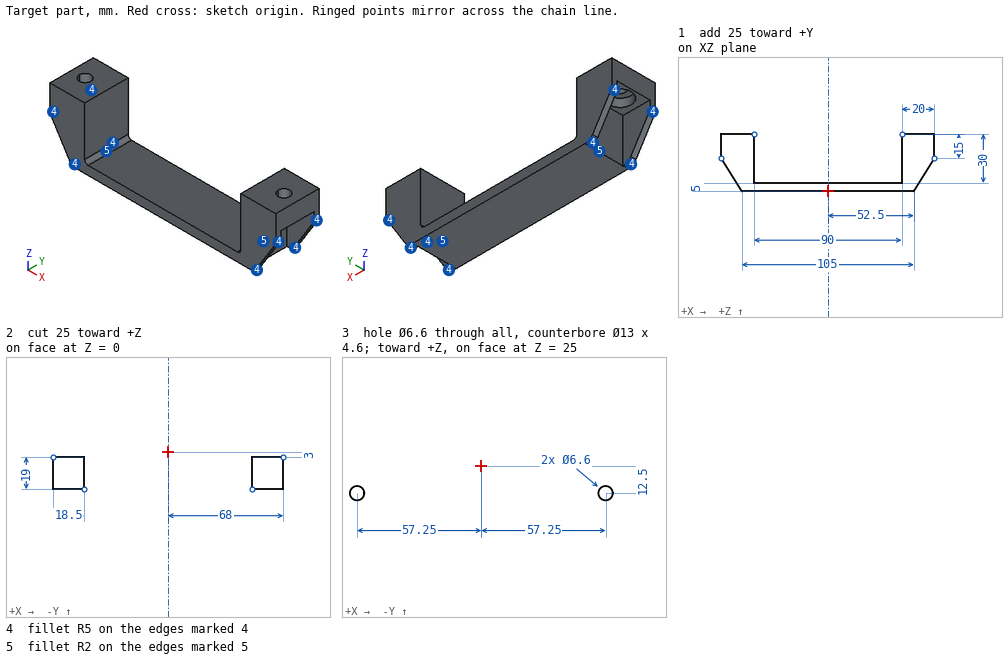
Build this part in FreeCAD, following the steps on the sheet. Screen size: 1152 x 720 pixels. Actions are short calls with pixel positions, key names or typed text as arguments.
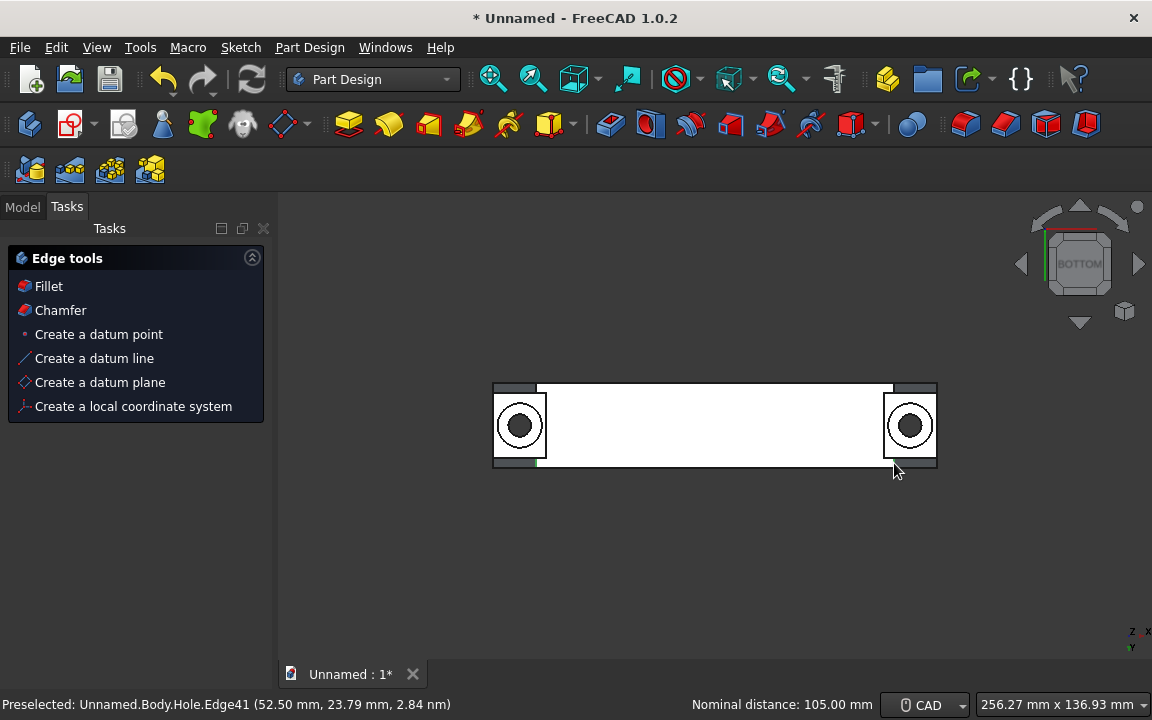
click(894, 388, ctrl)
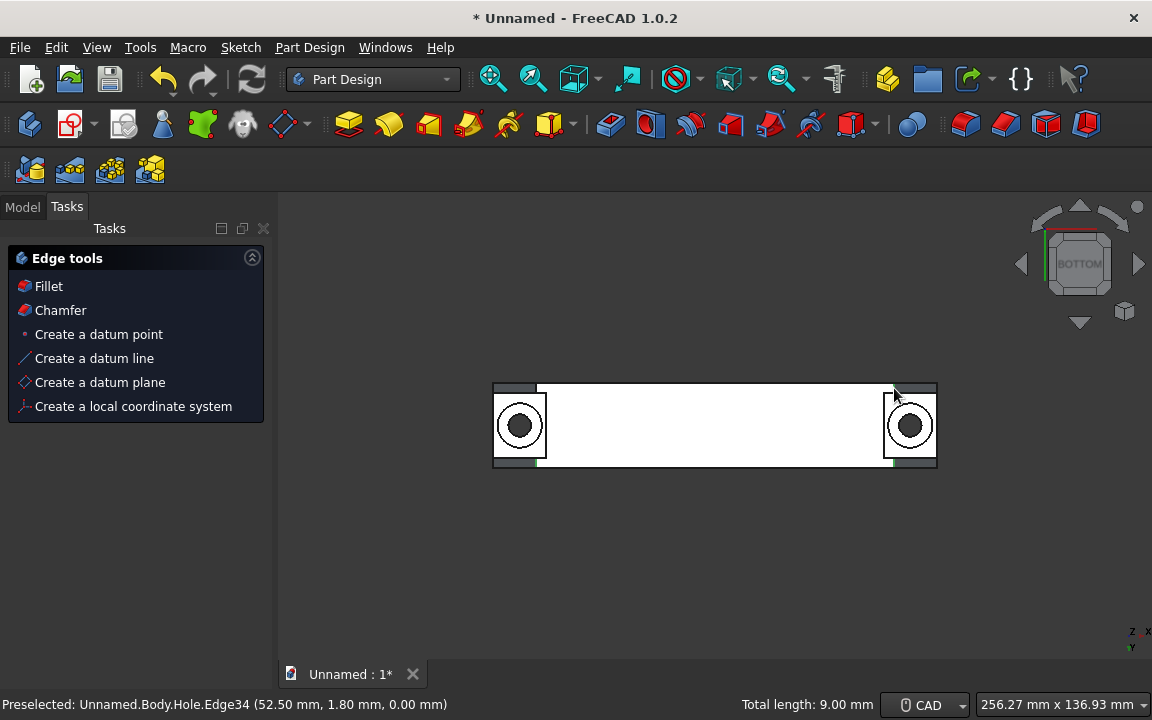
click(536, 388, ctrl)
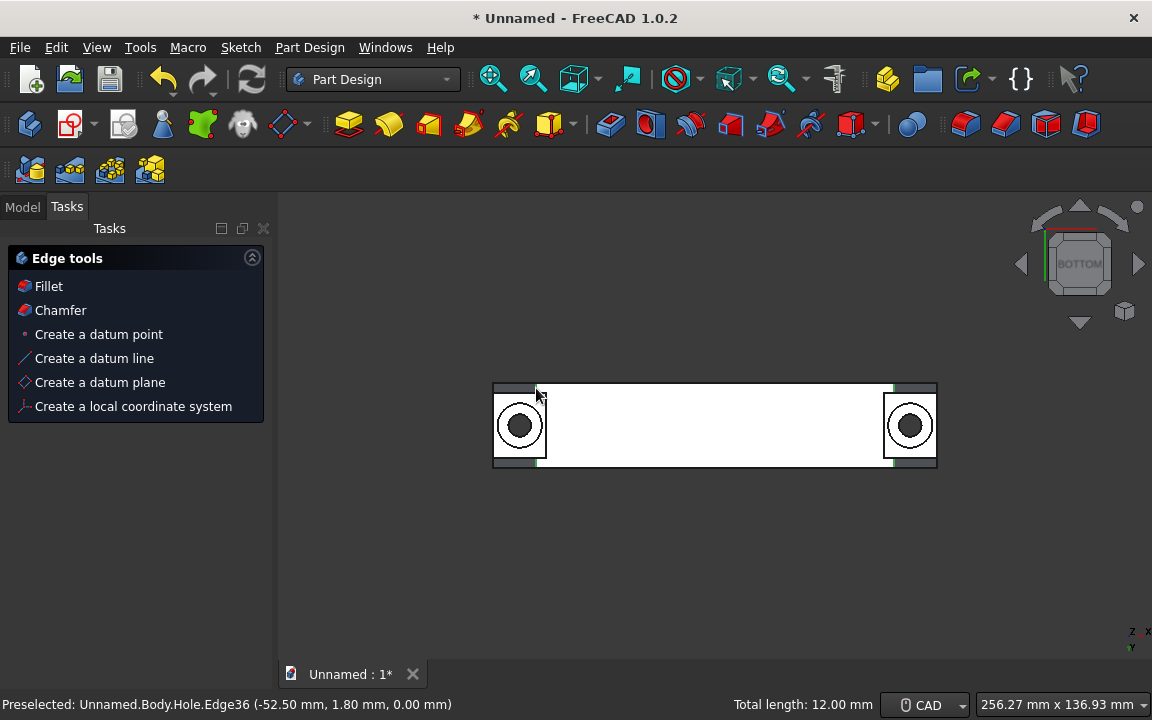
scroll(937, 462, up, 7)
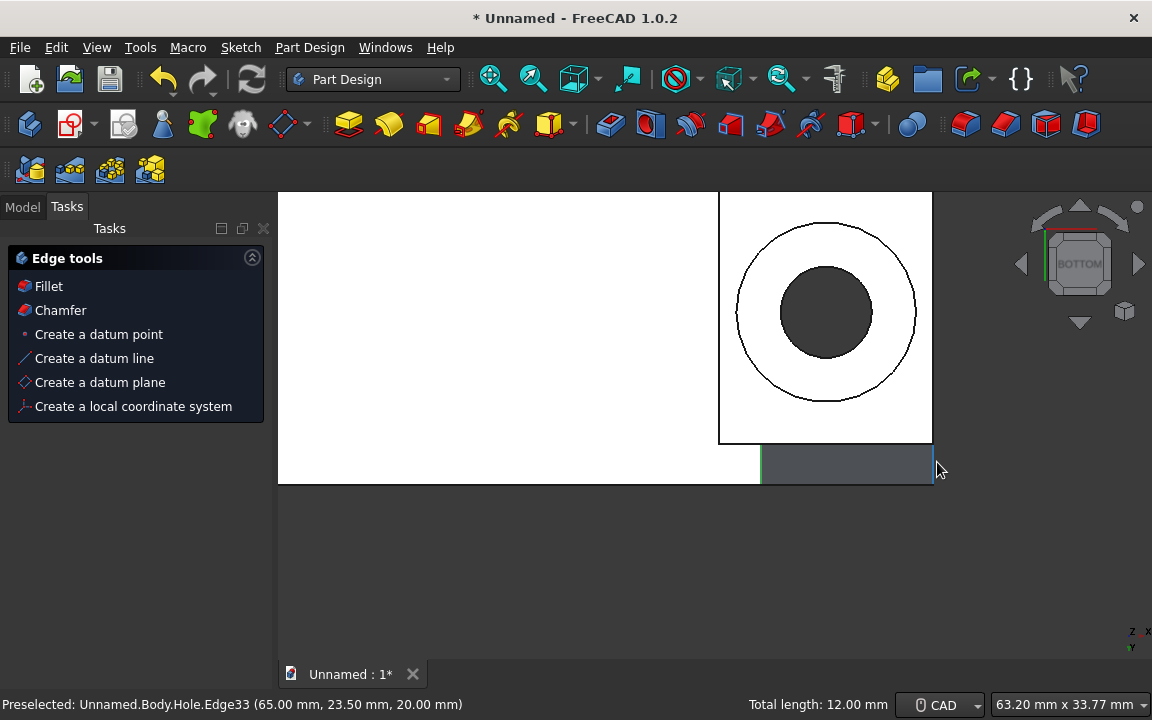
click(494, 80)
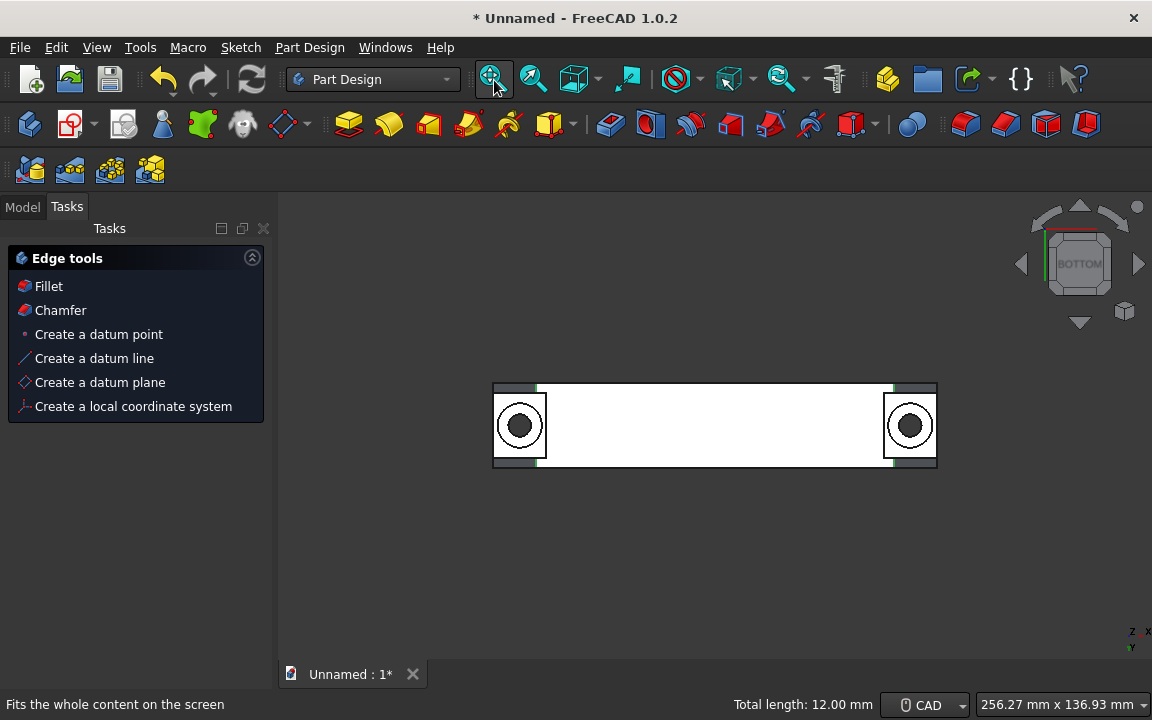
key(0)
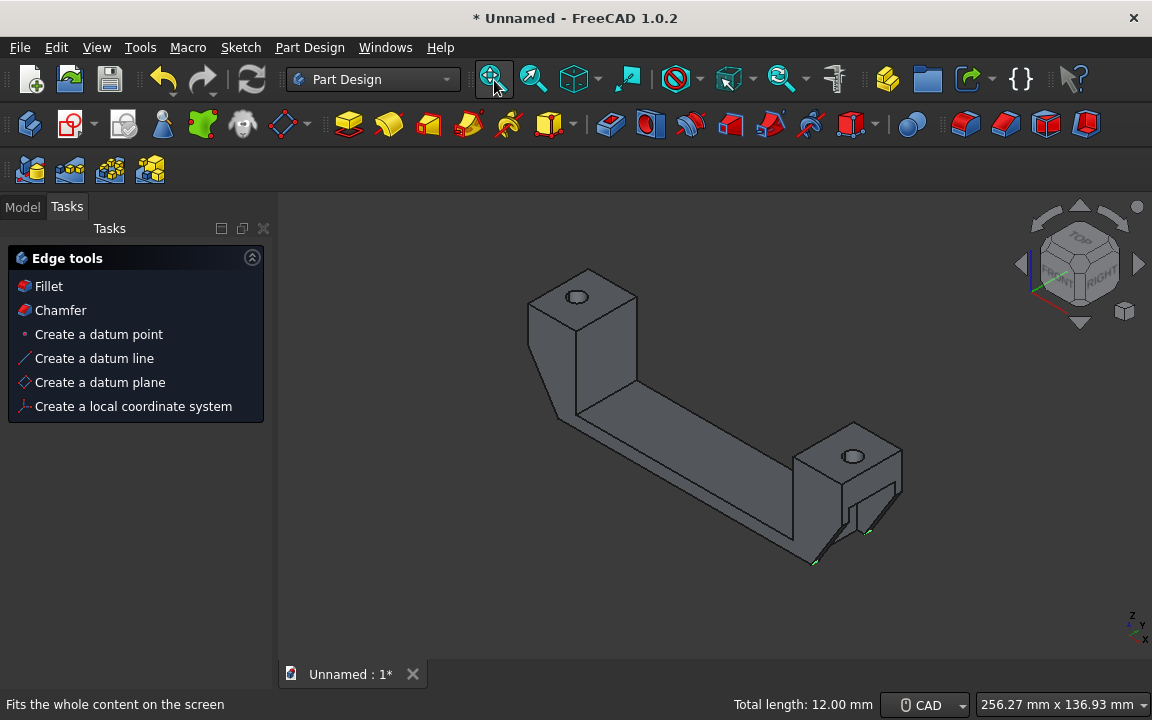
scroll(898, 493, up, 7)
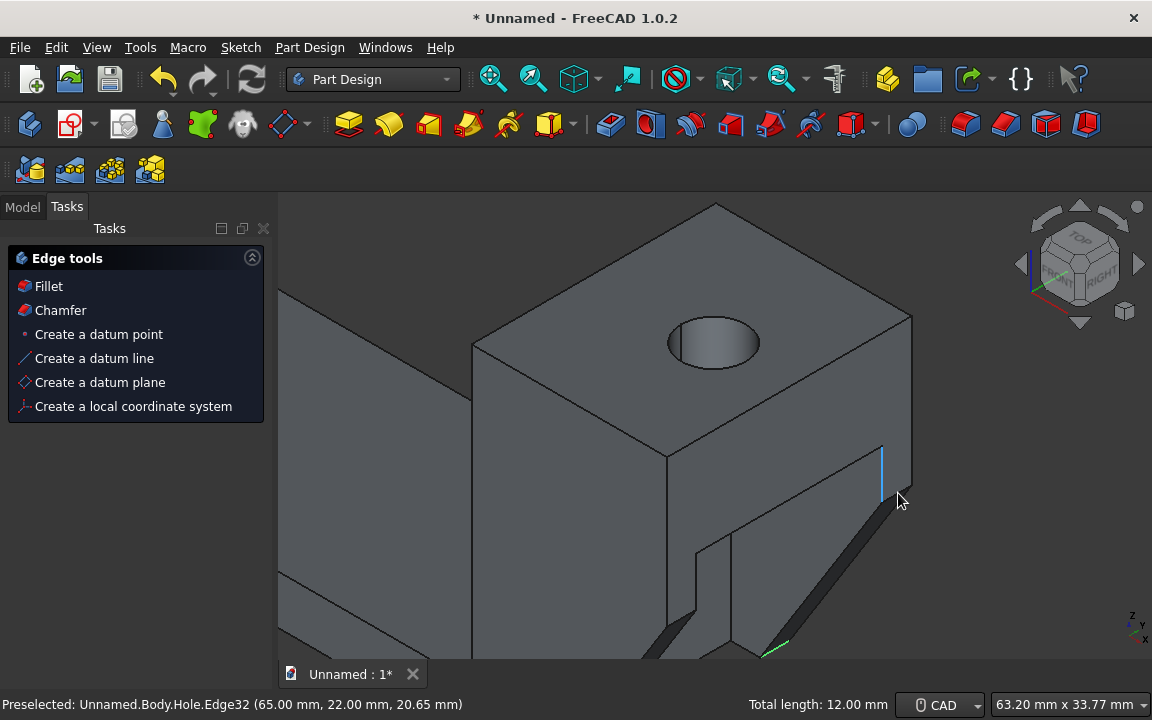
click(494, 80)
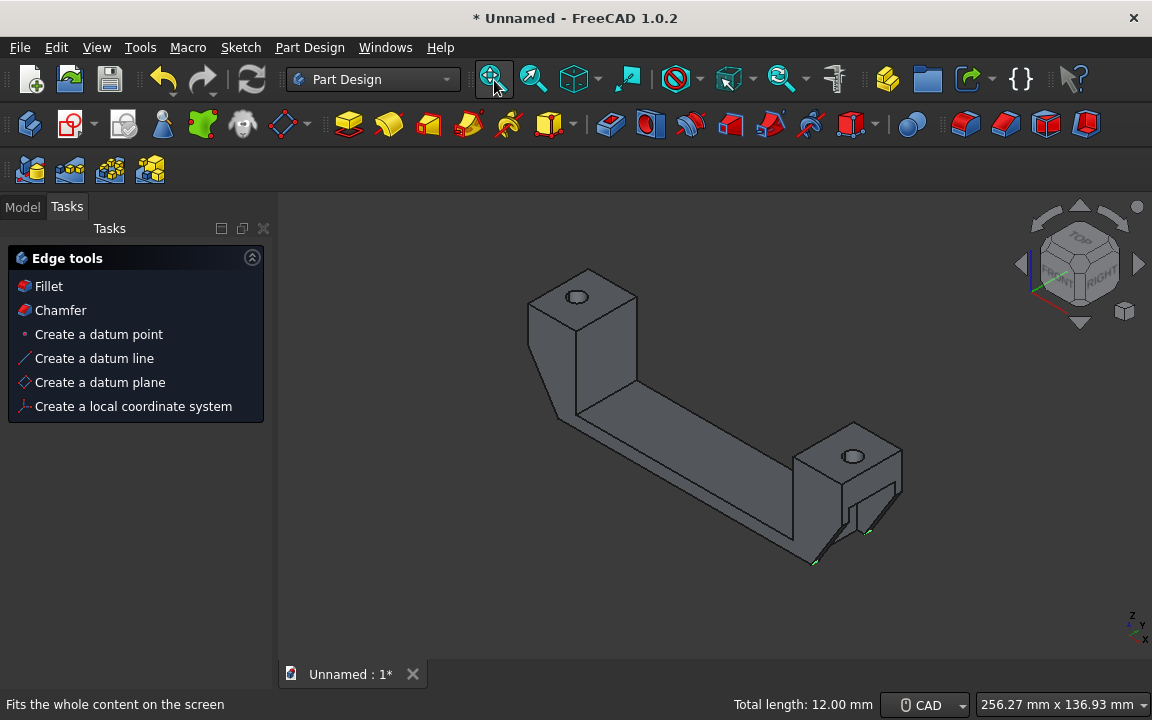
key(2)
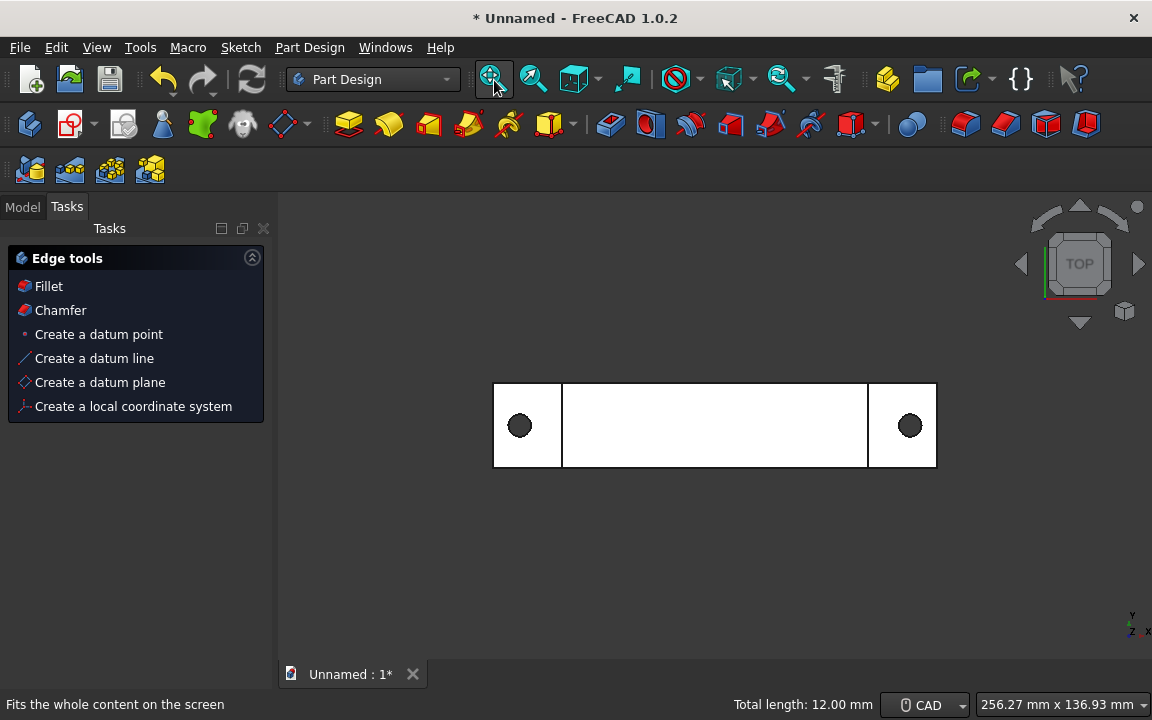
scroll(937, 387, up, 7)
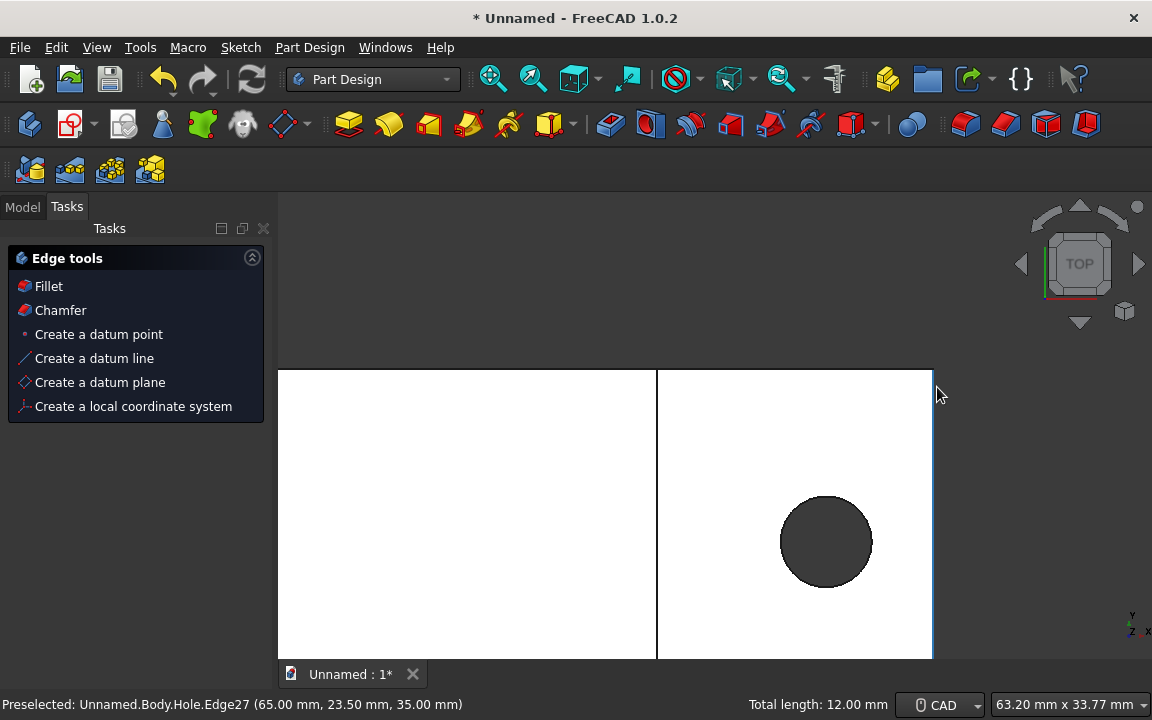
click(494, 80)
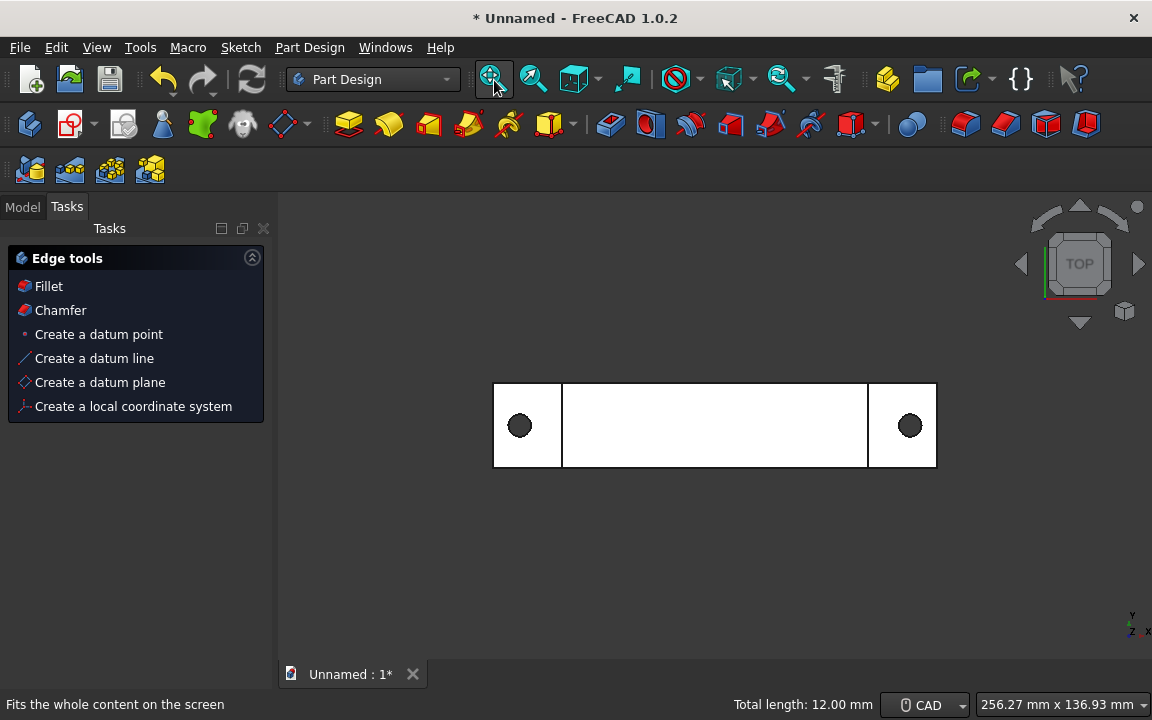
key(1)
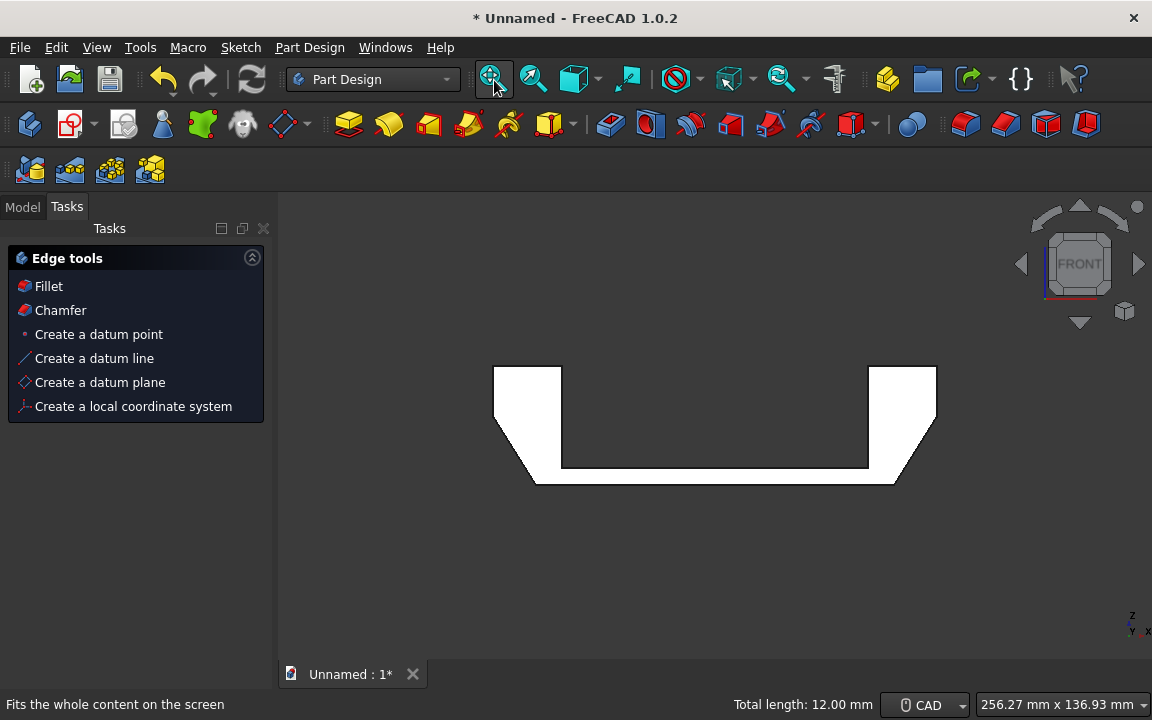
scroll(937, 416, up, 7)